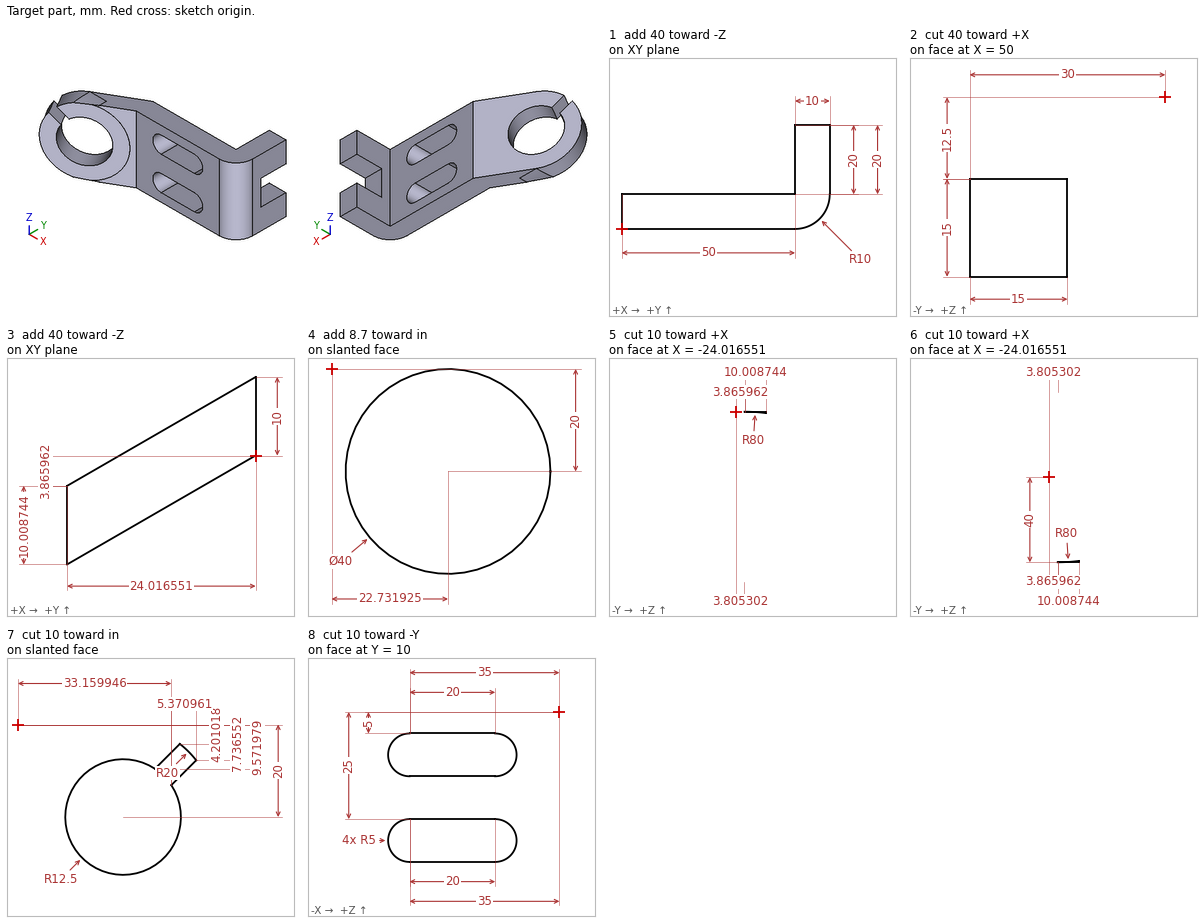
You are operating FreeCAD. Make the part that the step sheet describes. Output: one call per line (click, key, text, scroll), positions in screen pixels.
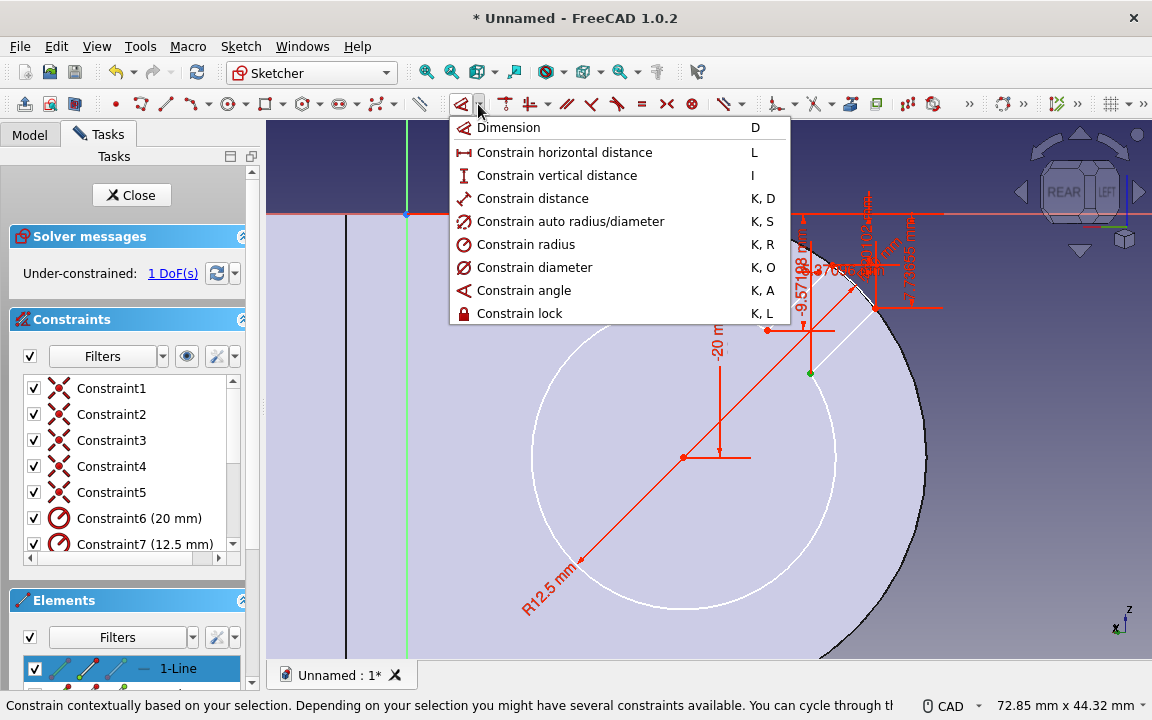
click(620, 152)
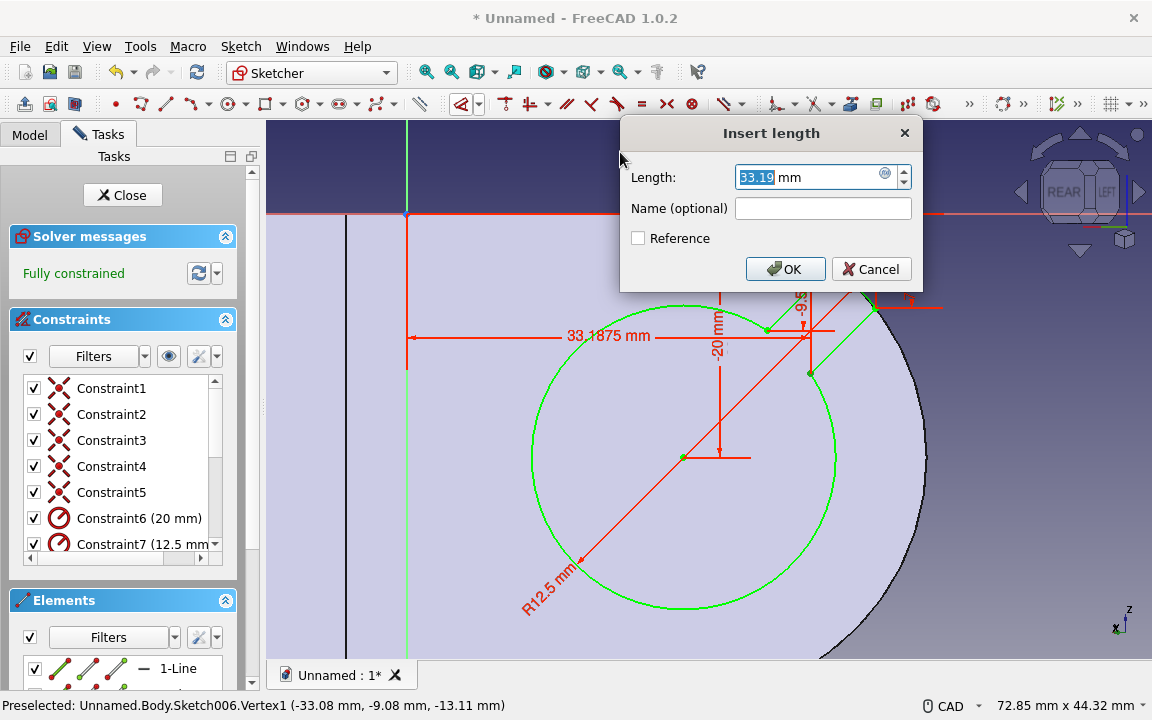
text(33.159946)
key(Return)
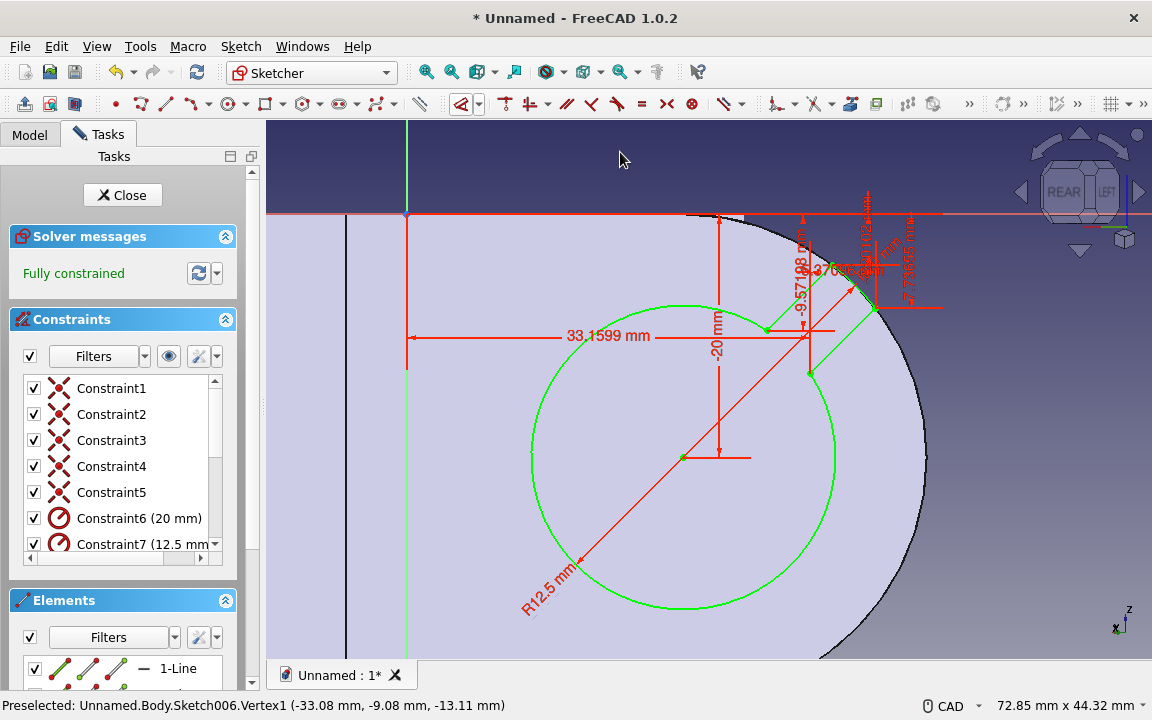
click(123, 195)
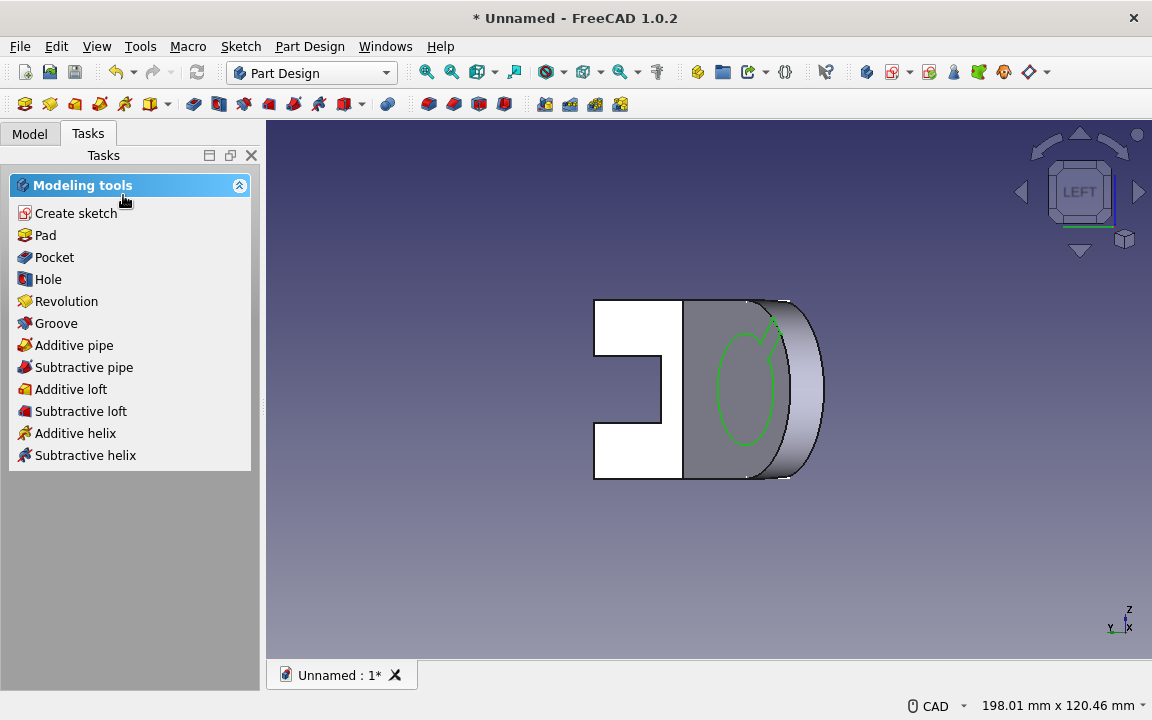
click(194, 104)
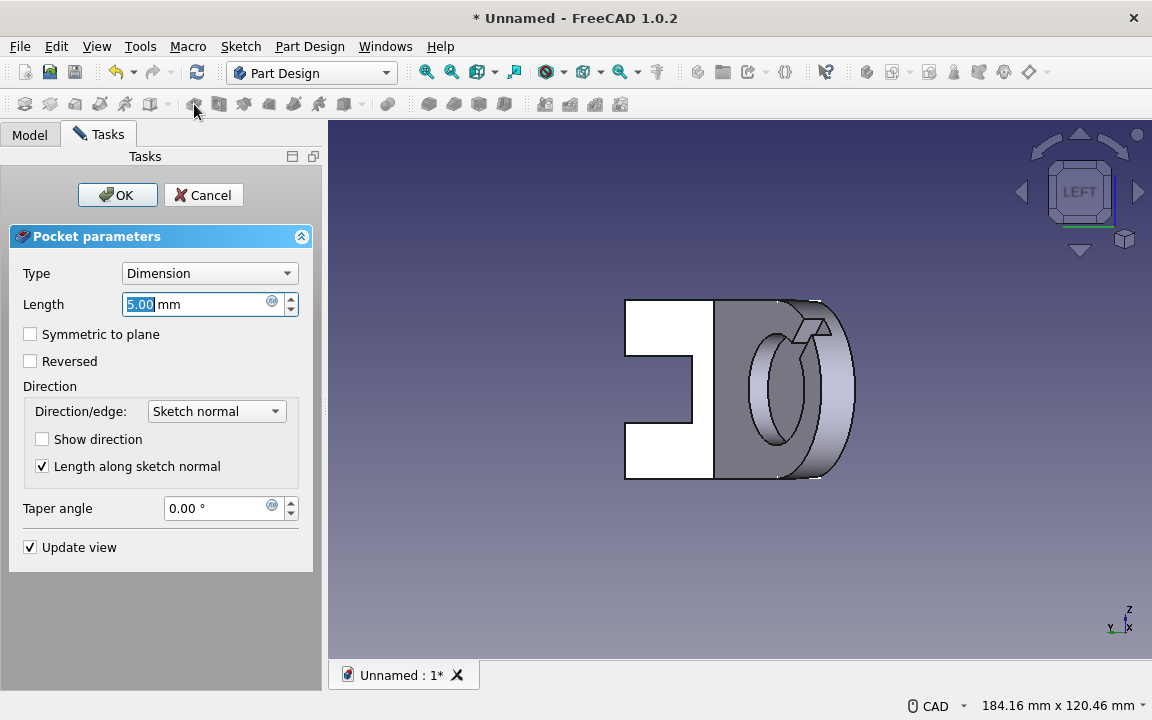
text(10)
key(Tab)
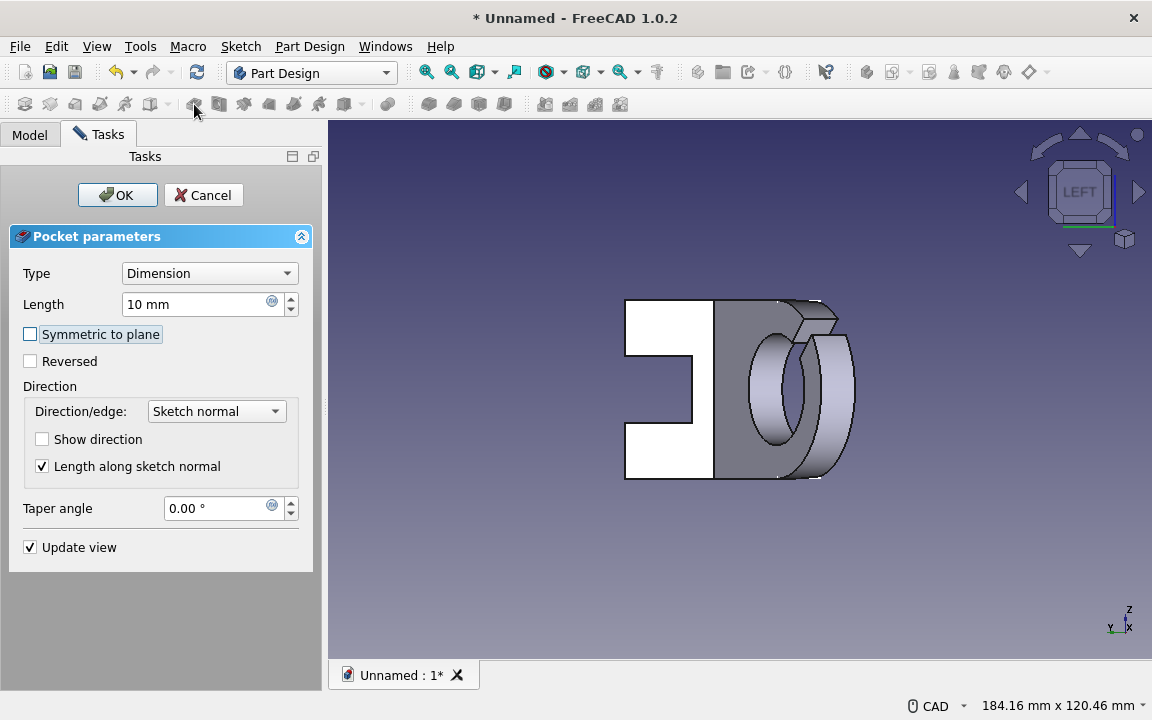
click(118, 195)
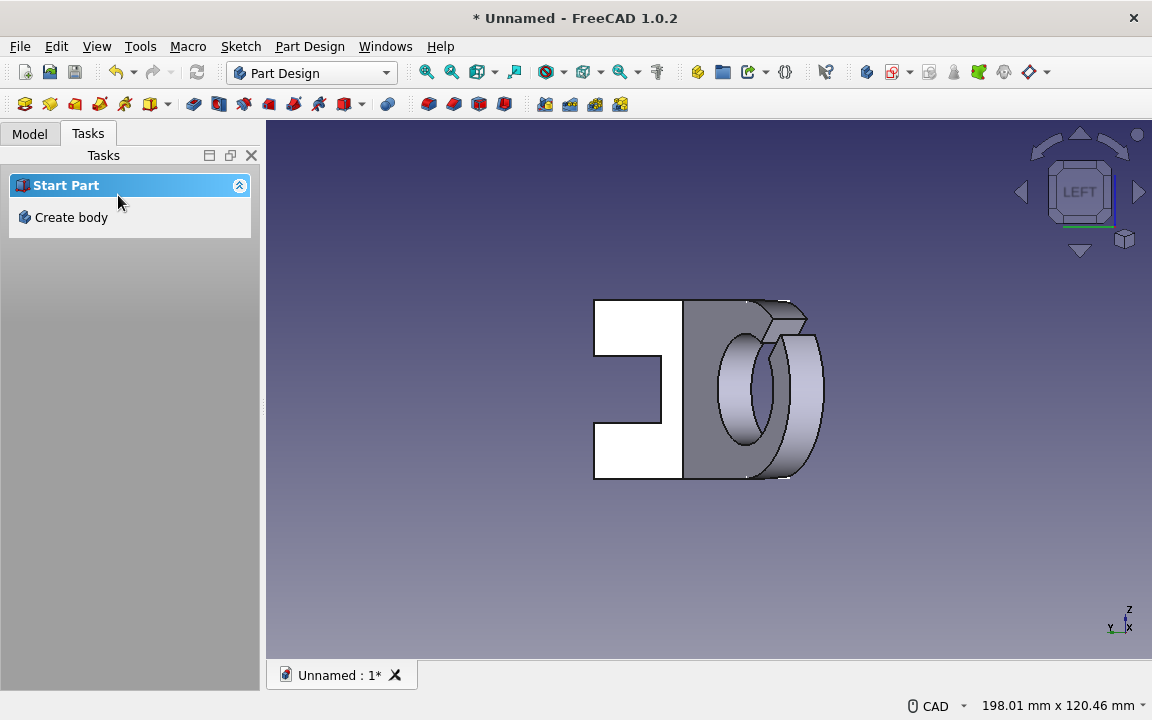
key(v)
key(f)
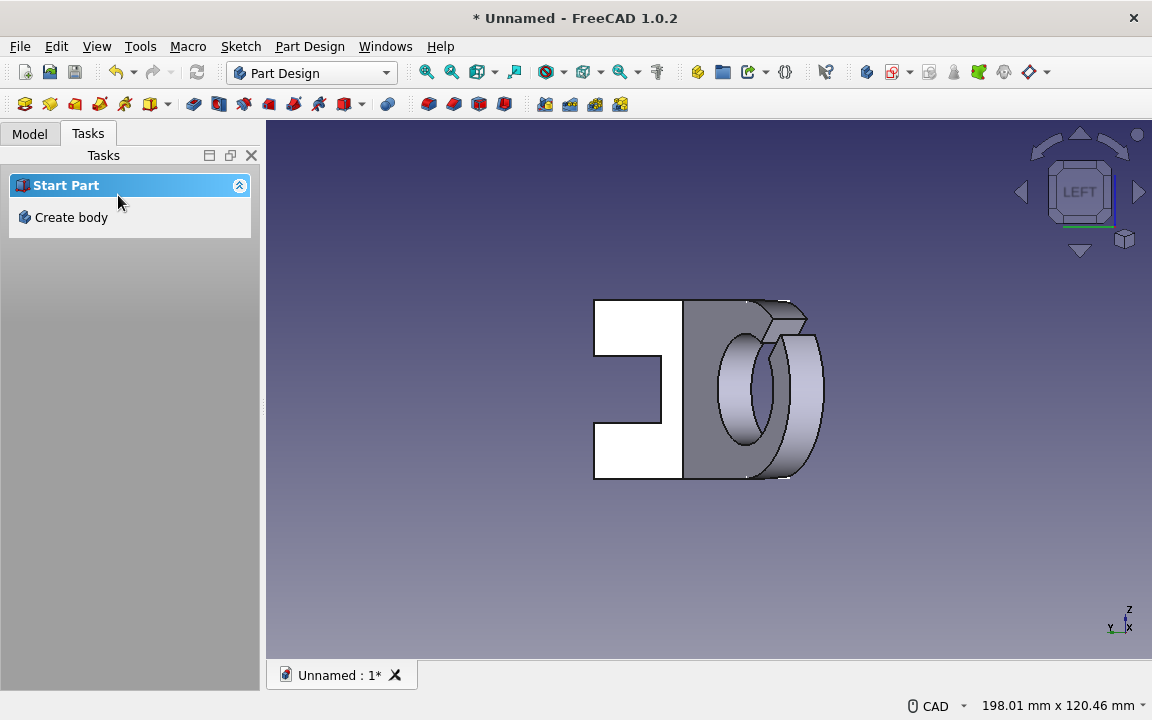
key(4)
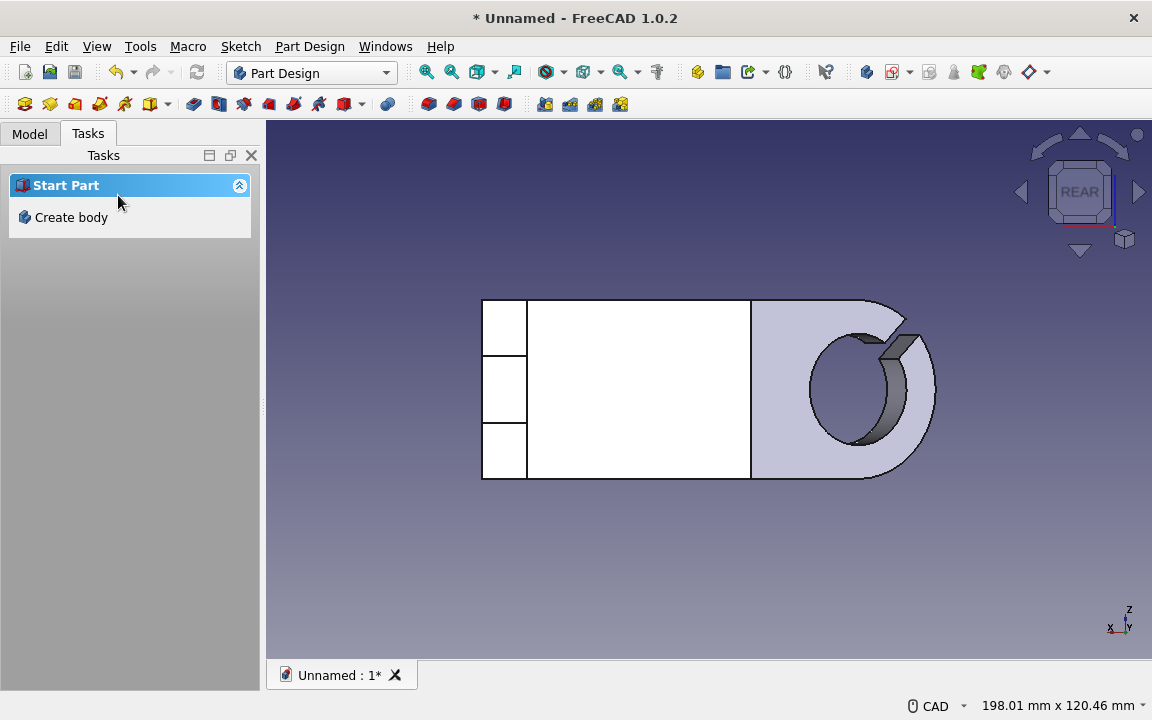
click(639, 388)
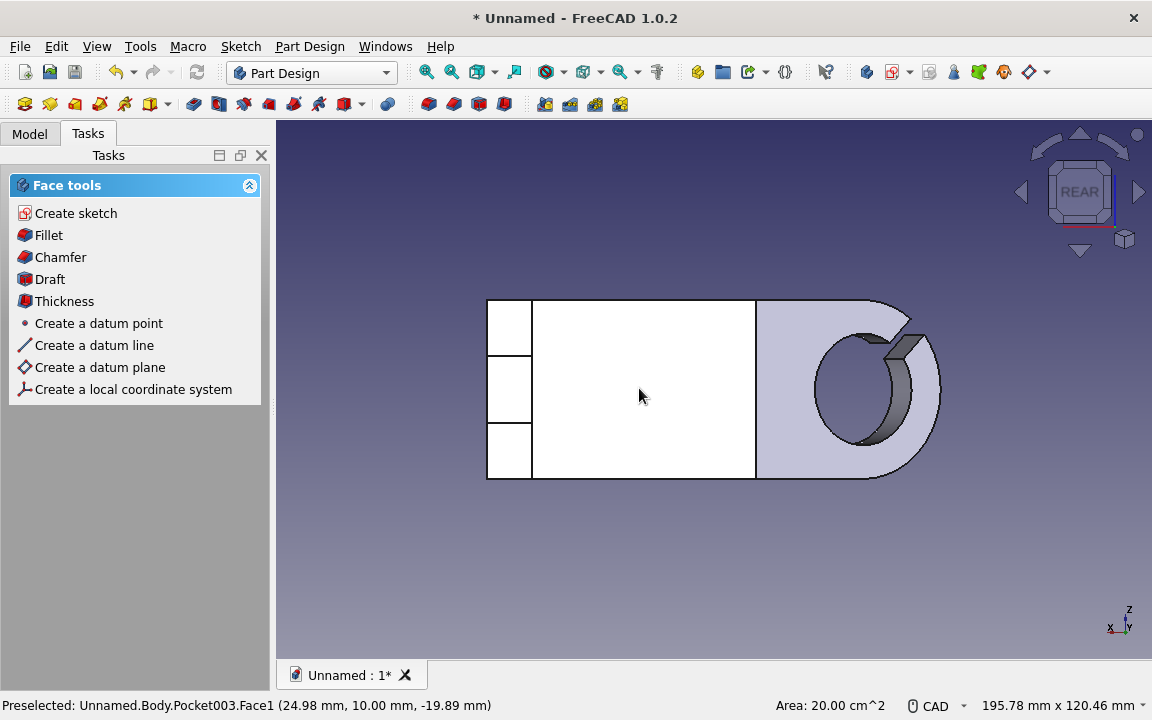
click(892, 72)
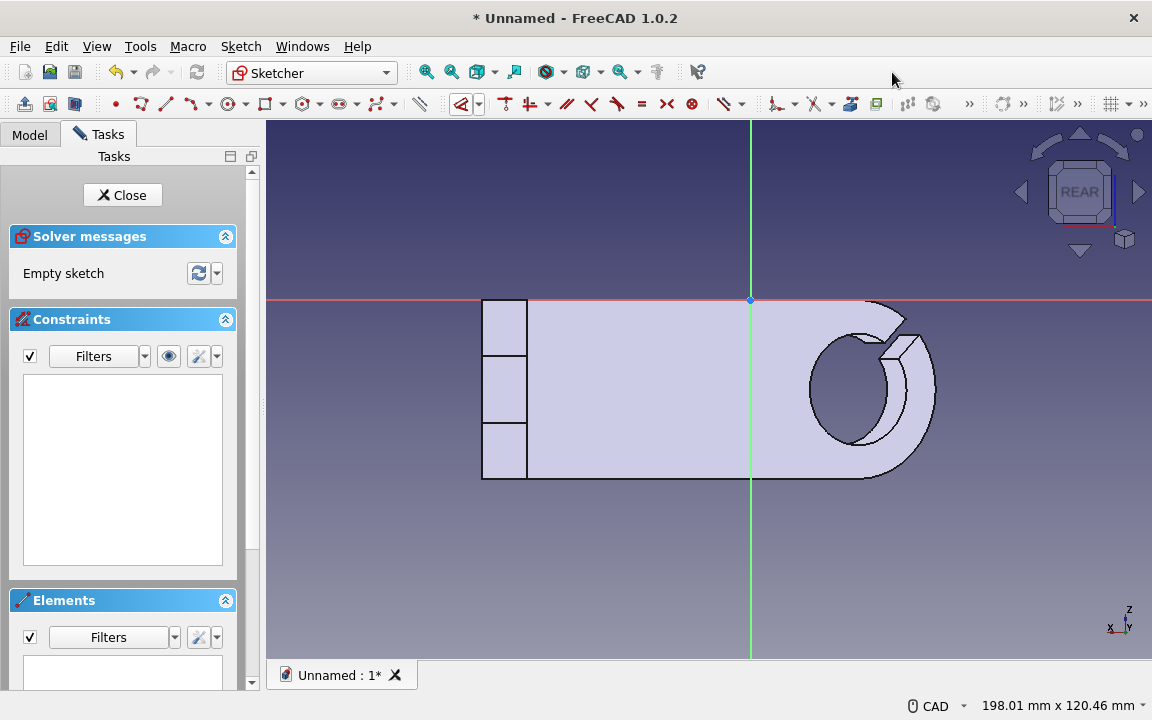
click(75, 104)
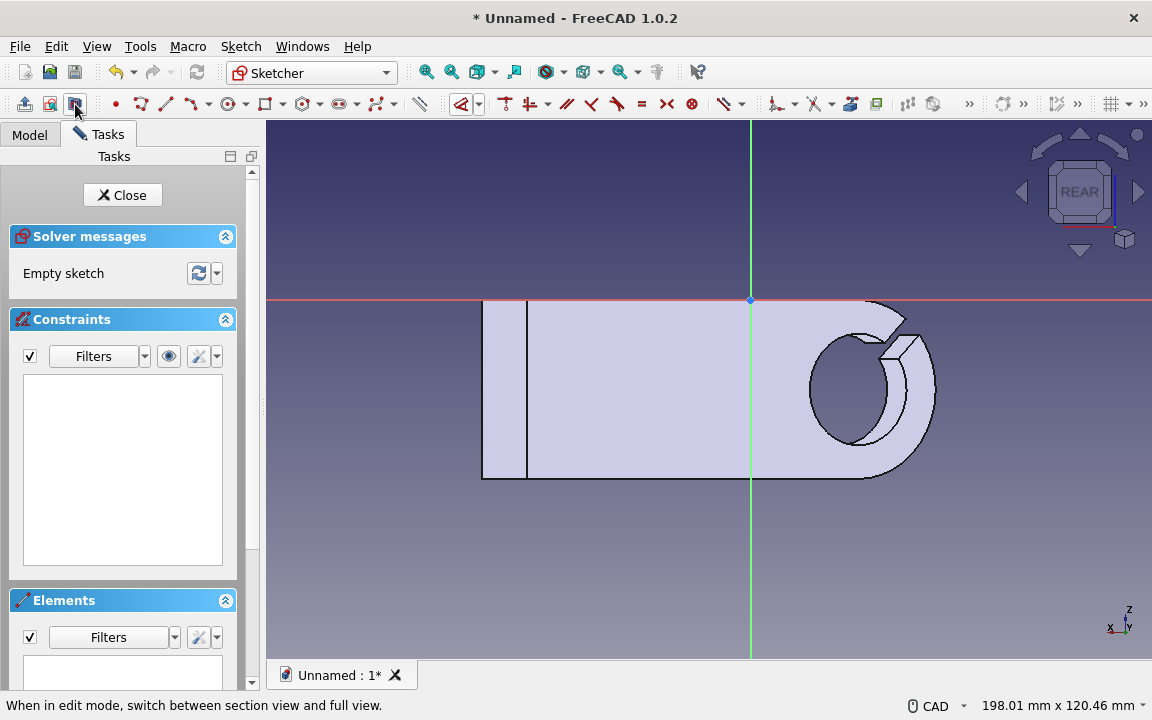
scroll(678, 369, up, 4)